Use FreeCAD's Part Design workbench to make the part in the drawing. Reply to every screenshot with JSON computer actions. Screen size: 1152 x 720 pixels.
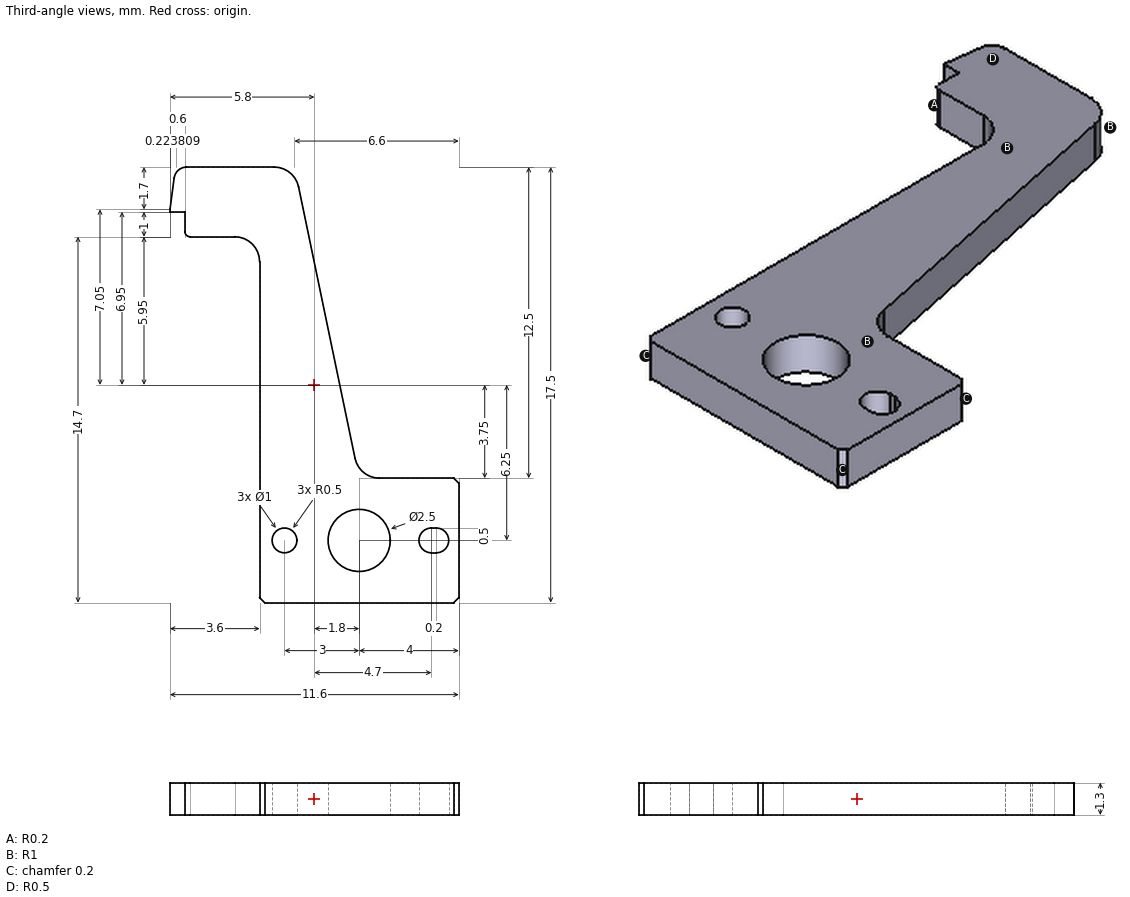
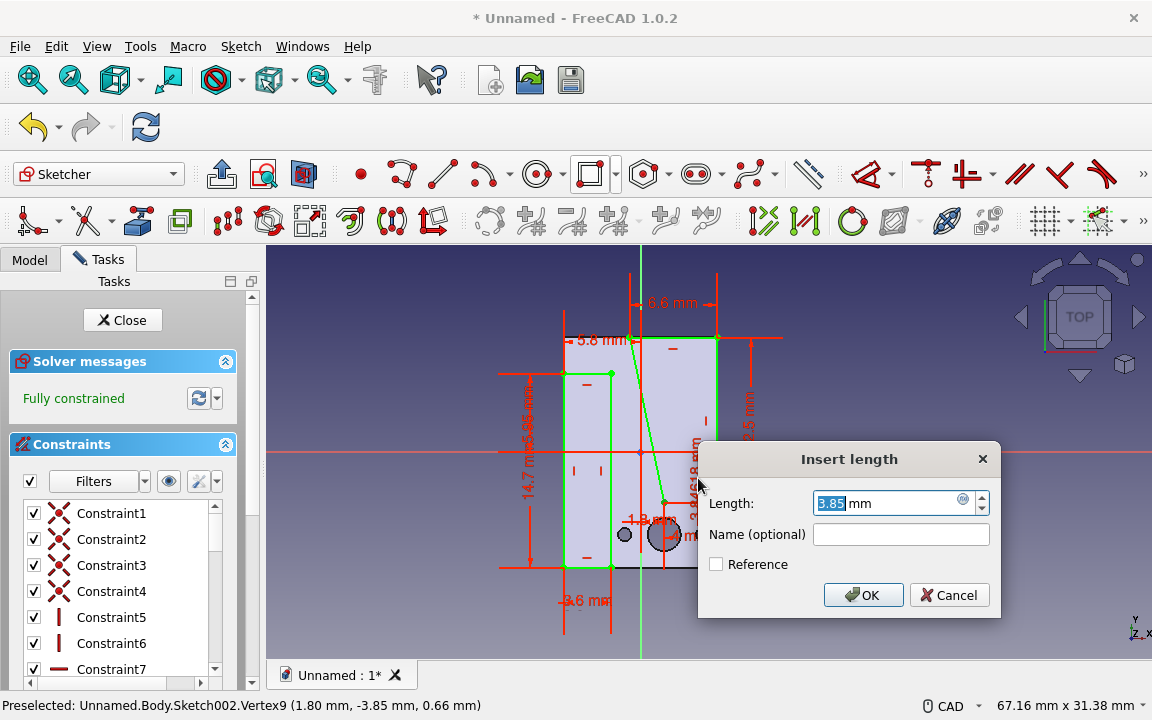
{"action": "type", "text": "3.75"}
{"action": "key", "text": "Return"}
{"action": "key", "text": "Escape"}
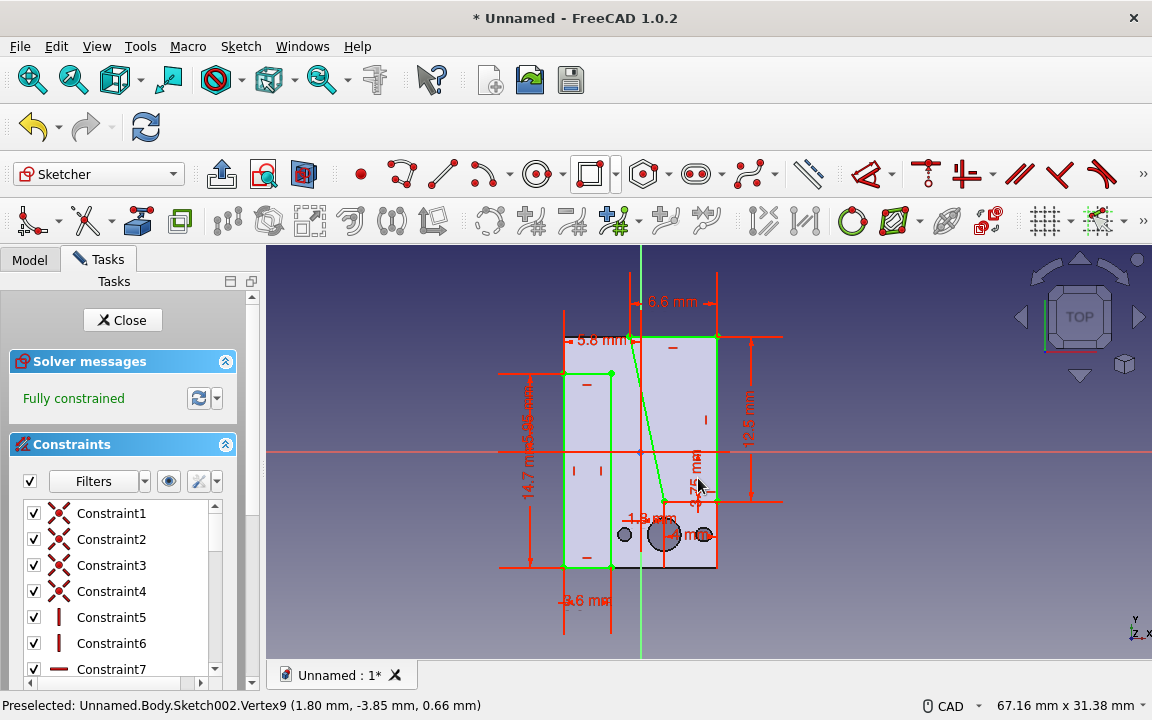
{"action": "left_click", "coordinate": [123, 320]}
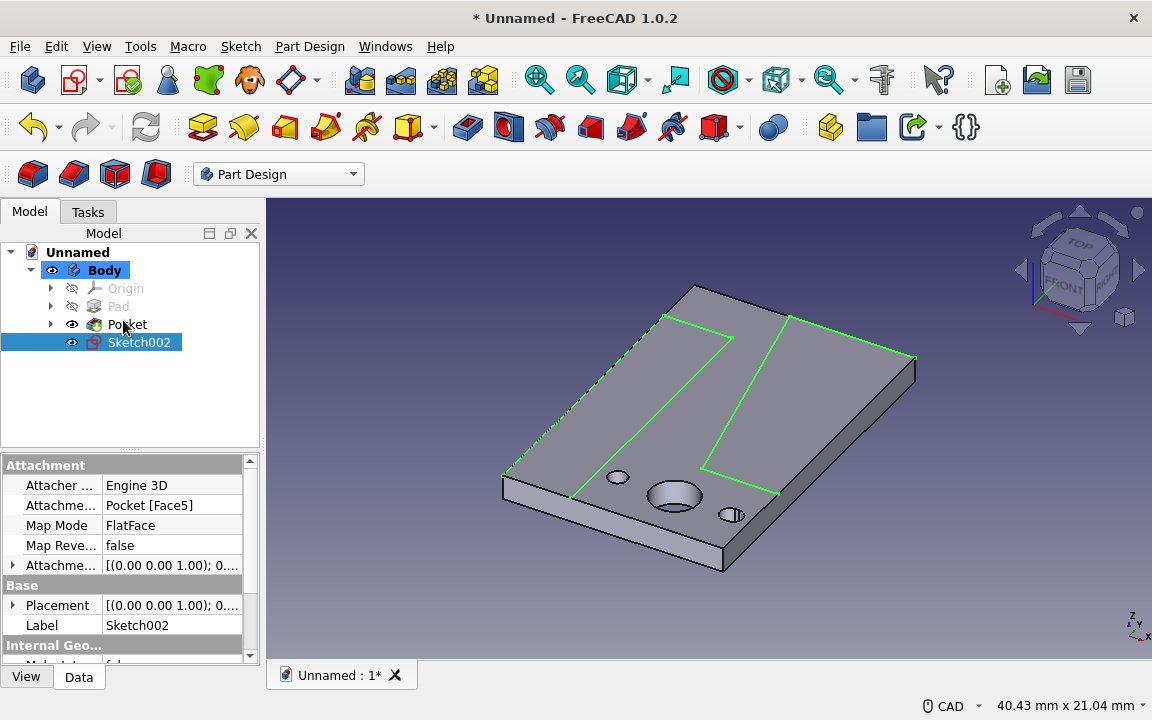
{"action": "left_click", "coordinate": [468, 128]}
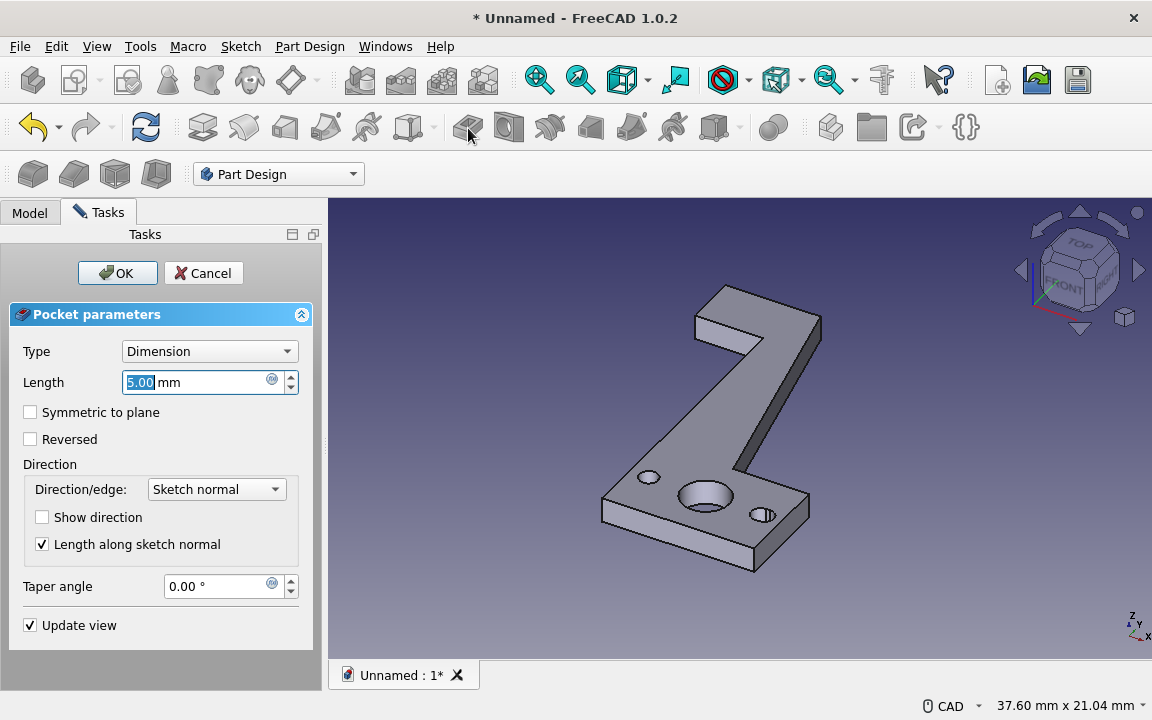
{"action": "left_click", "coordinate": [210, 352]}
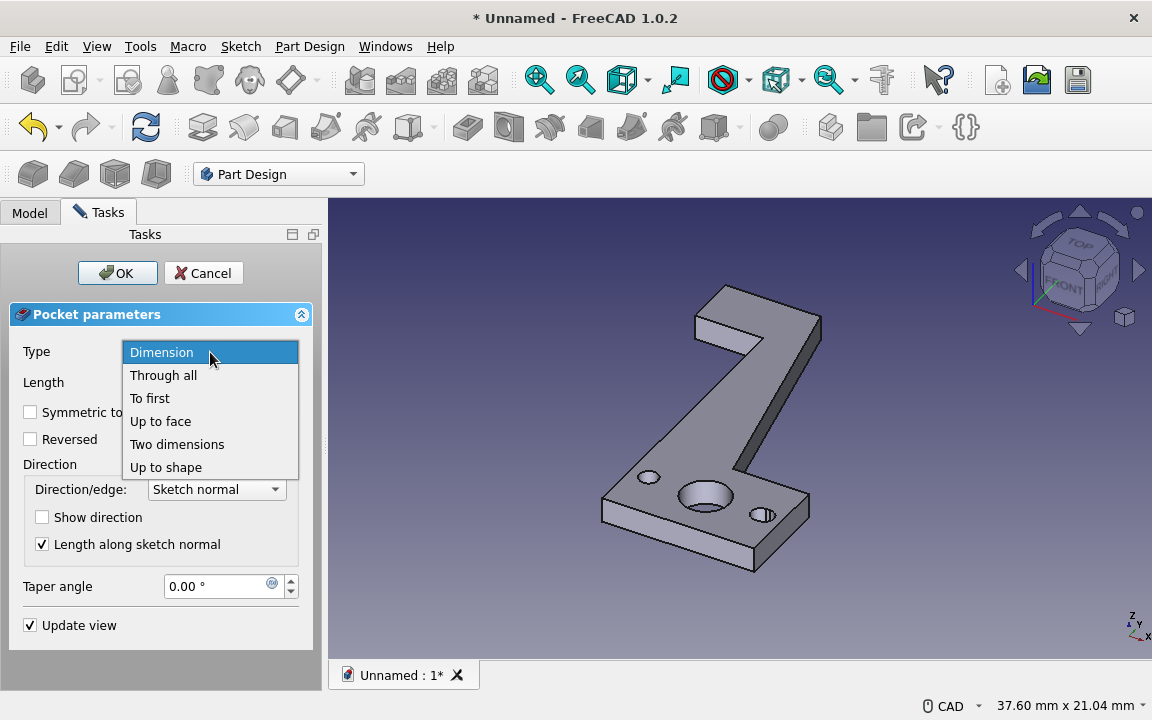
{"action": "left_click", "coordinate": [208, 376]}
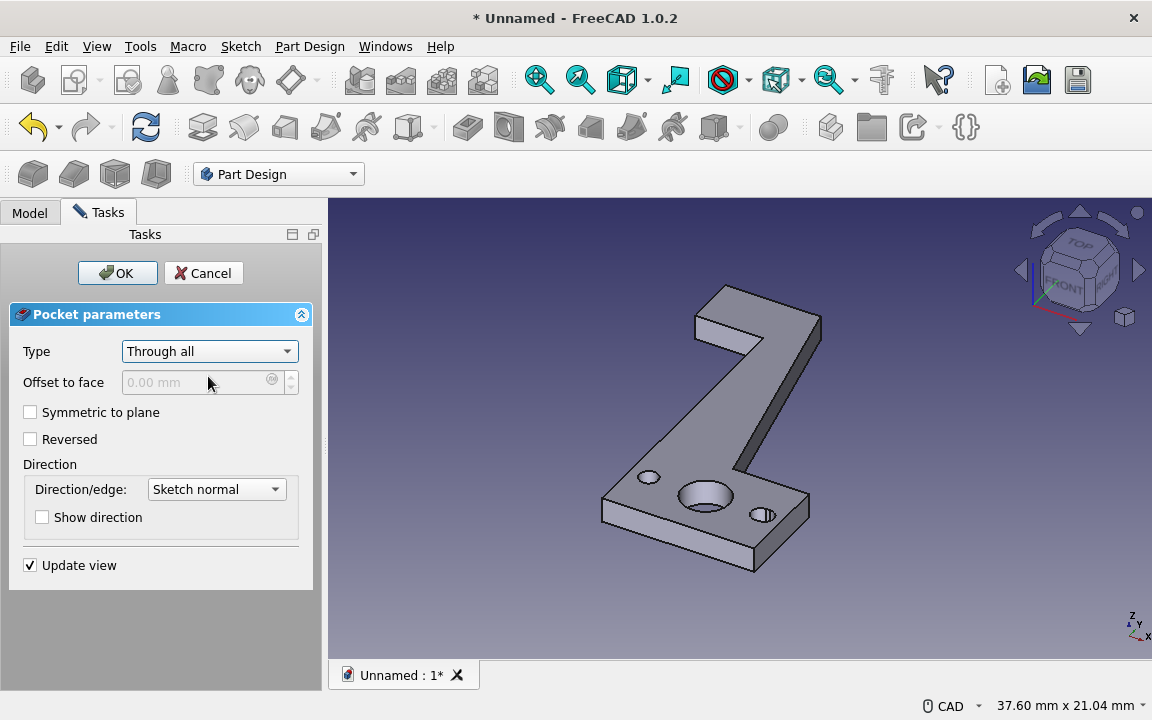
{"action": "left_click", "coordinate": [118, 273]}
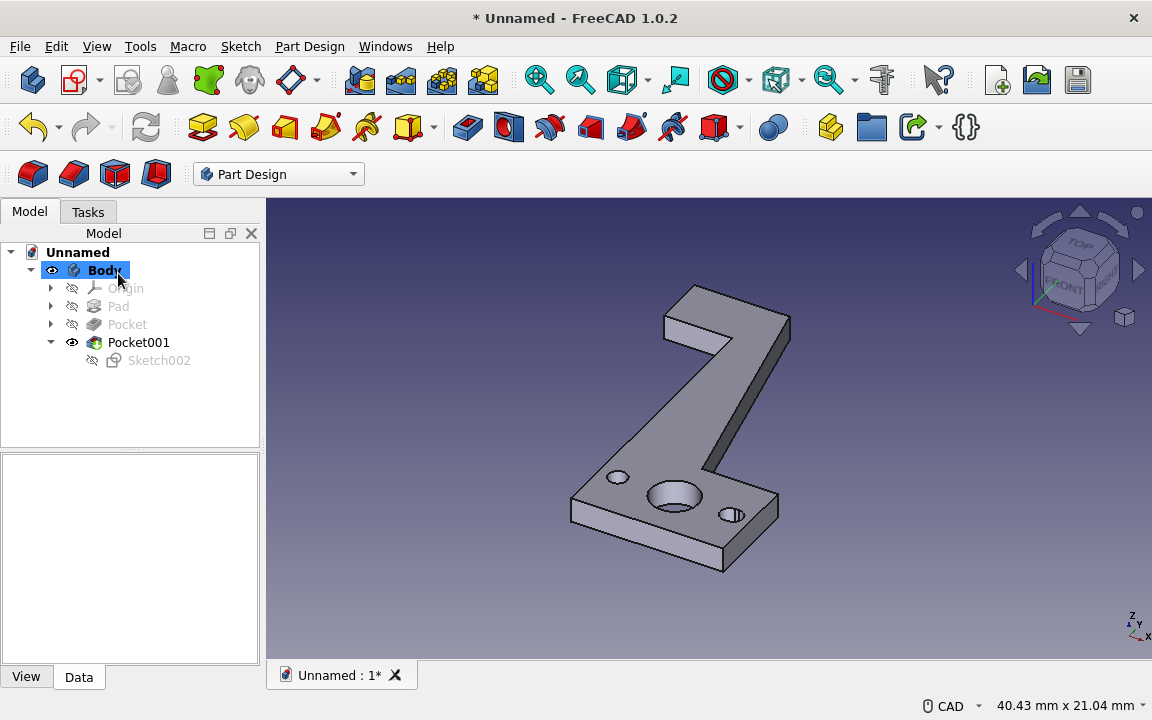
{"action": "left_click", "coordinate": [682, 443]}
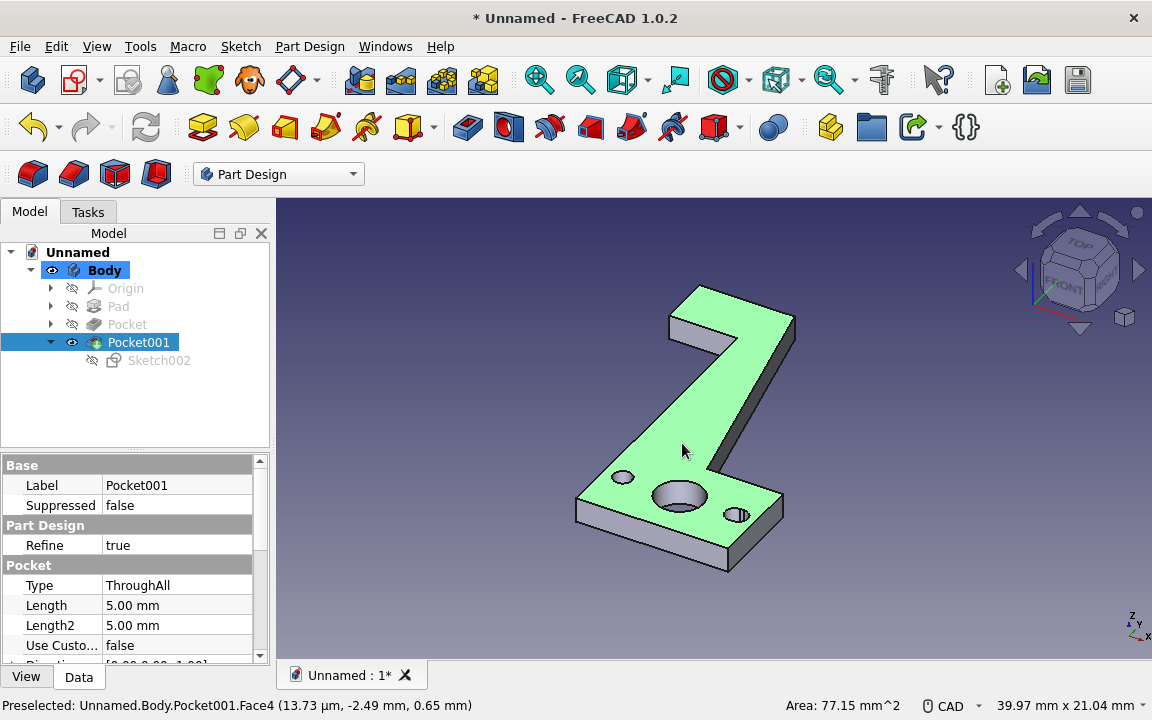
{"action": "left_click", "coordinate": [74, 80]}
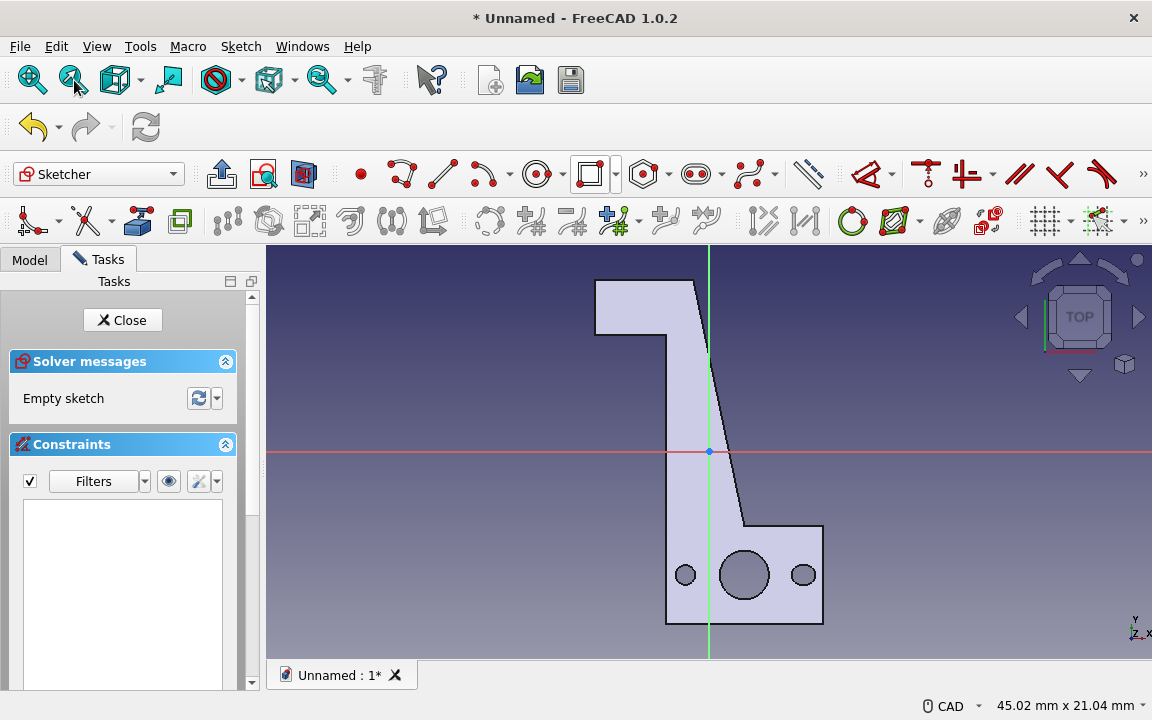
{"action": "scroll", "coordinate": [598, 315], "scroll_direction": "up", "scroll_amount": 13}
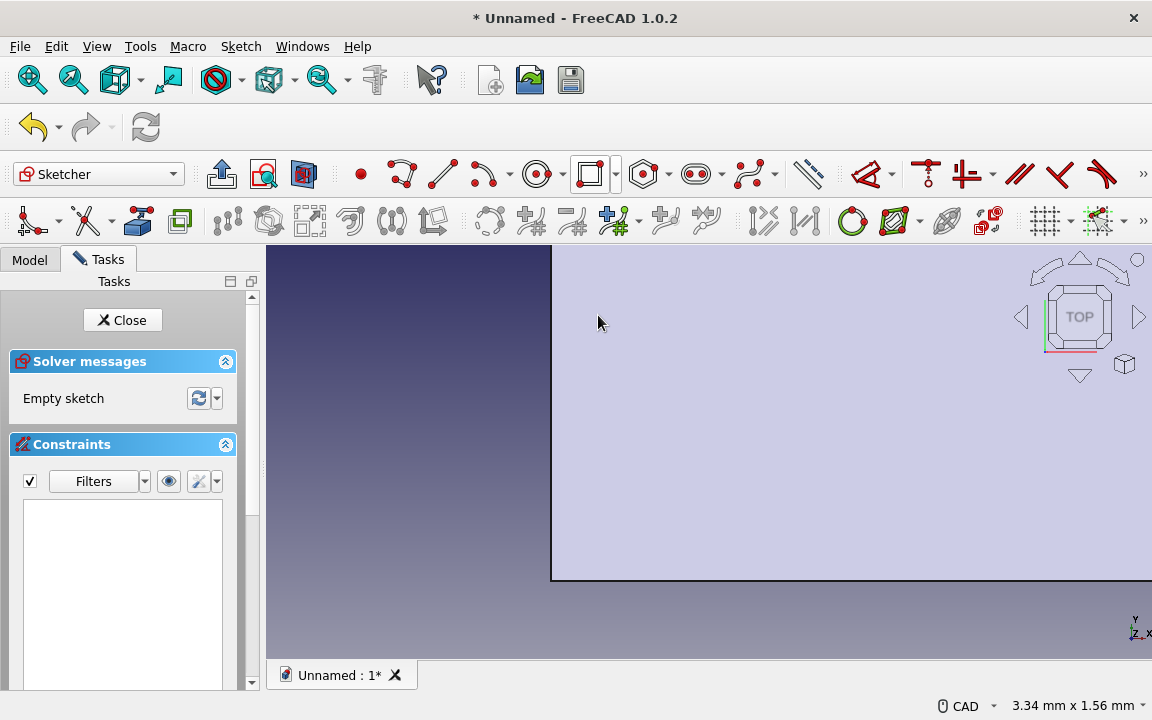
{"action": "key", "text": "g r"}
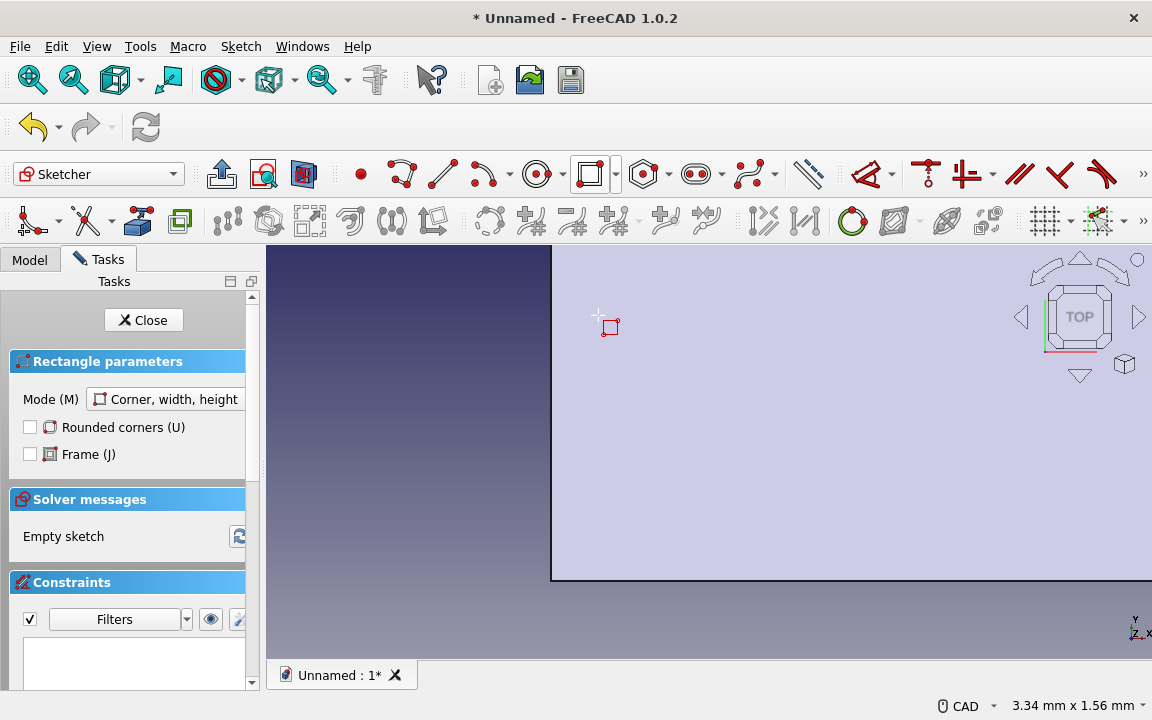
{"action": "left_click", "coordinate": [551, 316]}
{"action": "left_click", "coordinate": [710, 581]}
{"action": "key", "text": "Escape"}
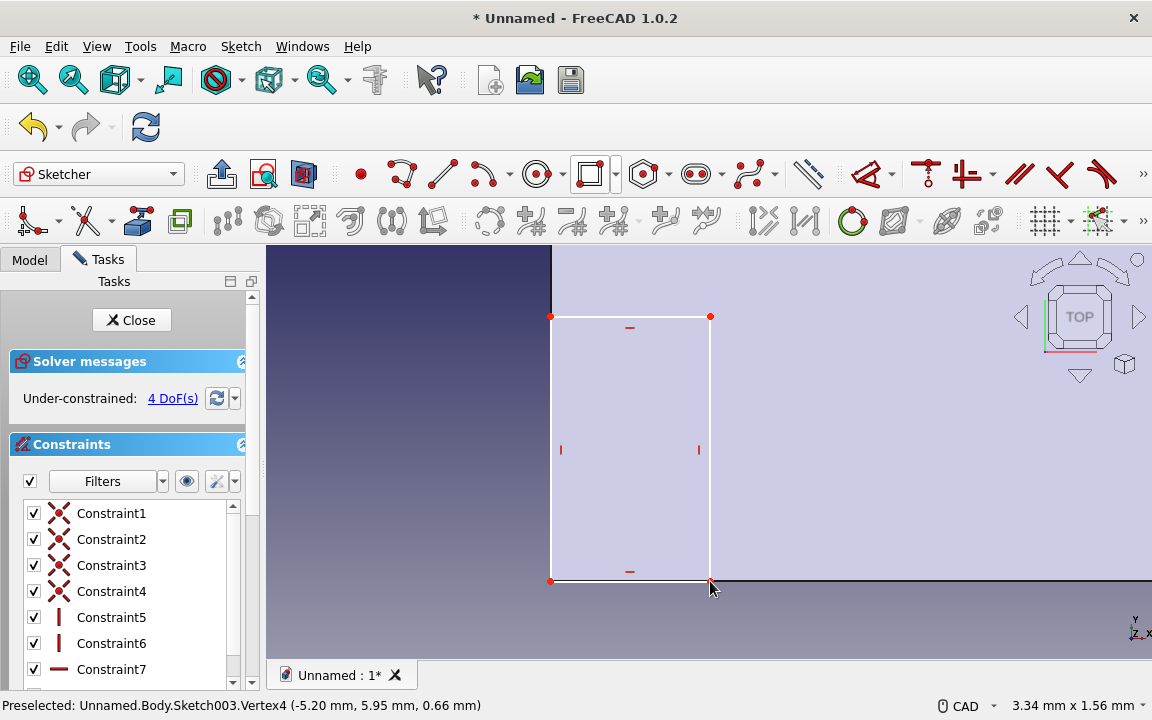
{"action": "key", "text": "d"}